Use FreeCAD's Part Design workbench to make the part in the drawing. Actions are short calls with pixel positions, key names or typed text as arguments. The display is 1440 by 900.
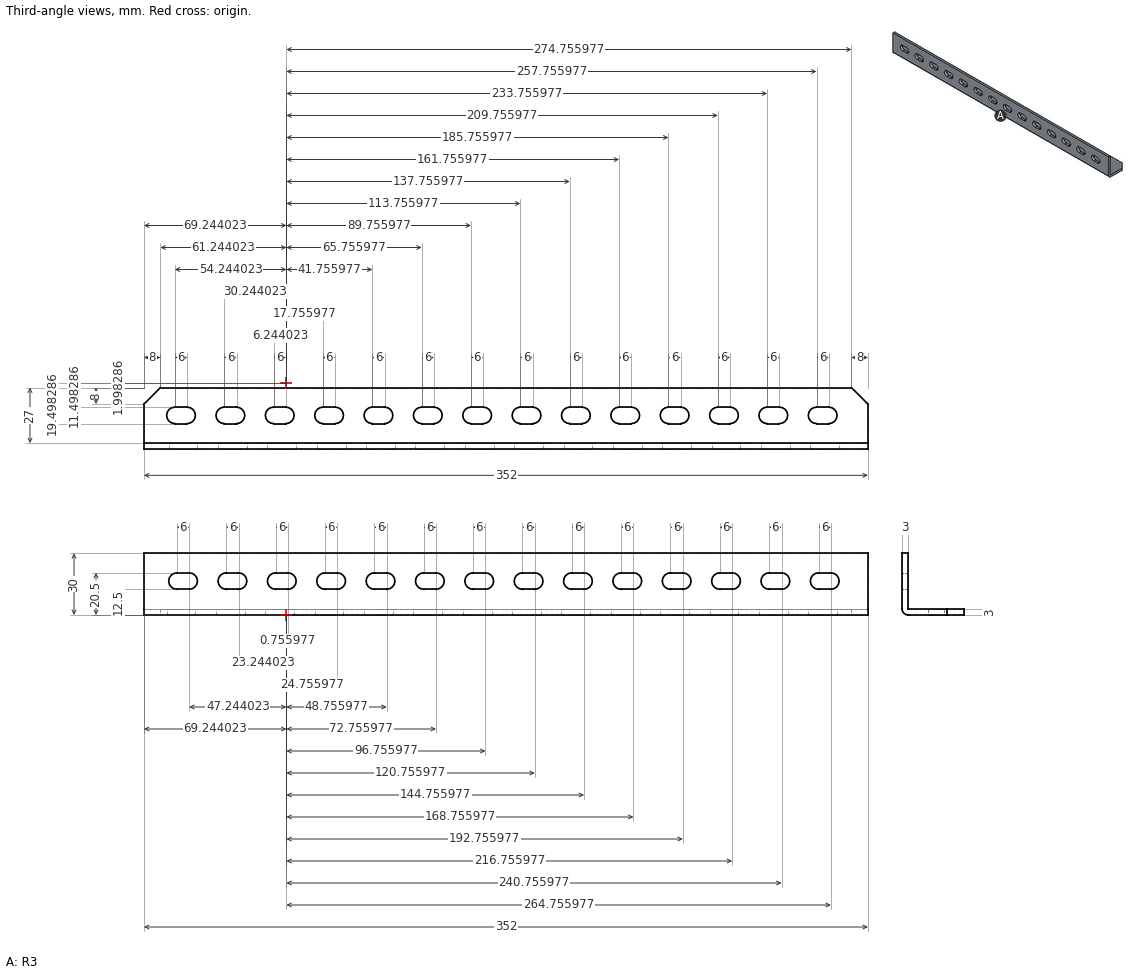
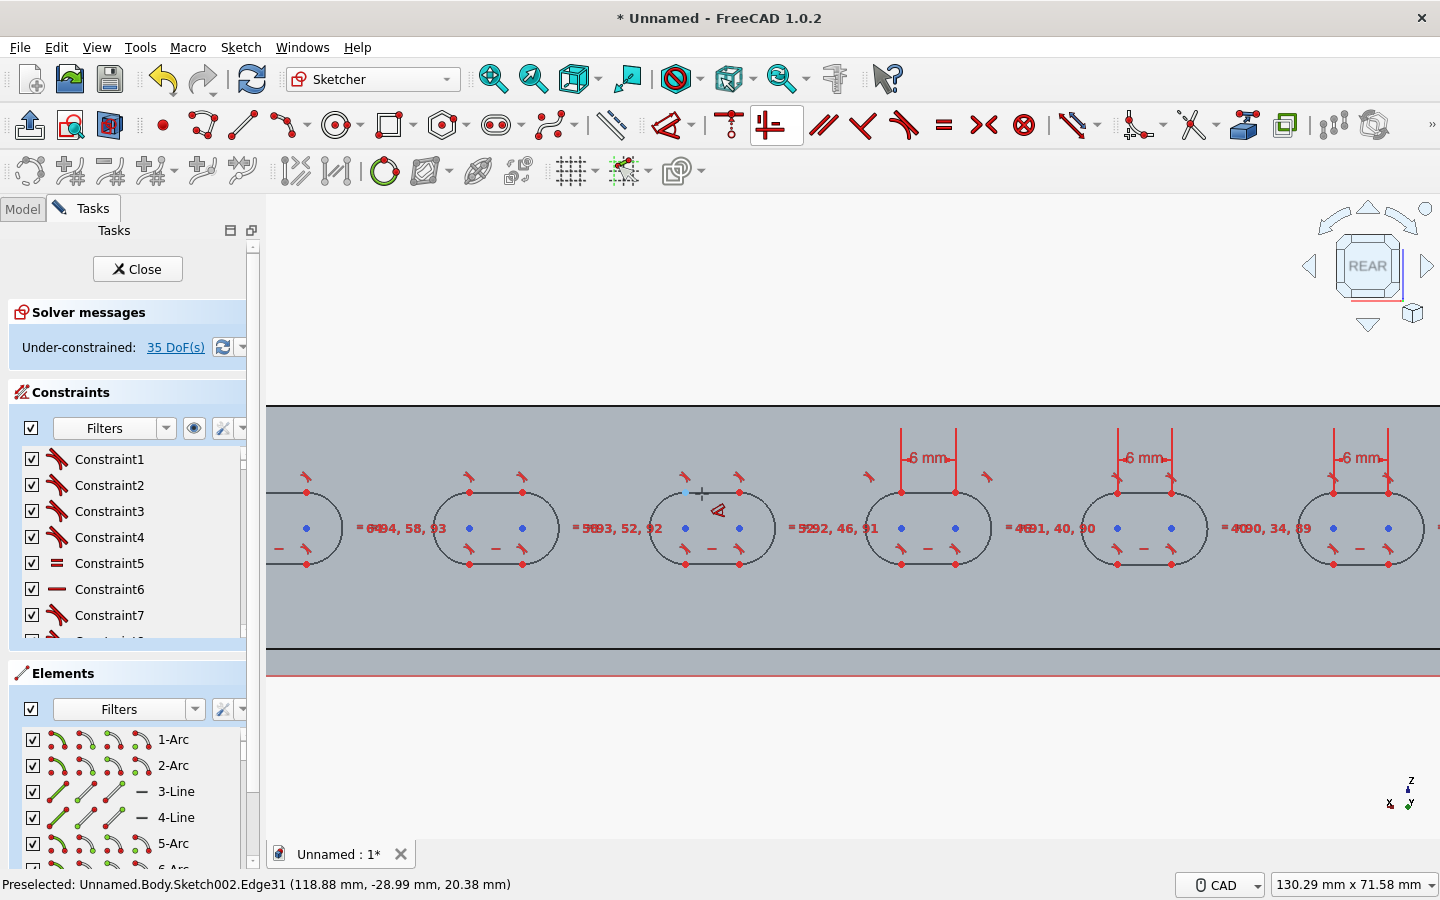
click(702, 493)
click(712, 459)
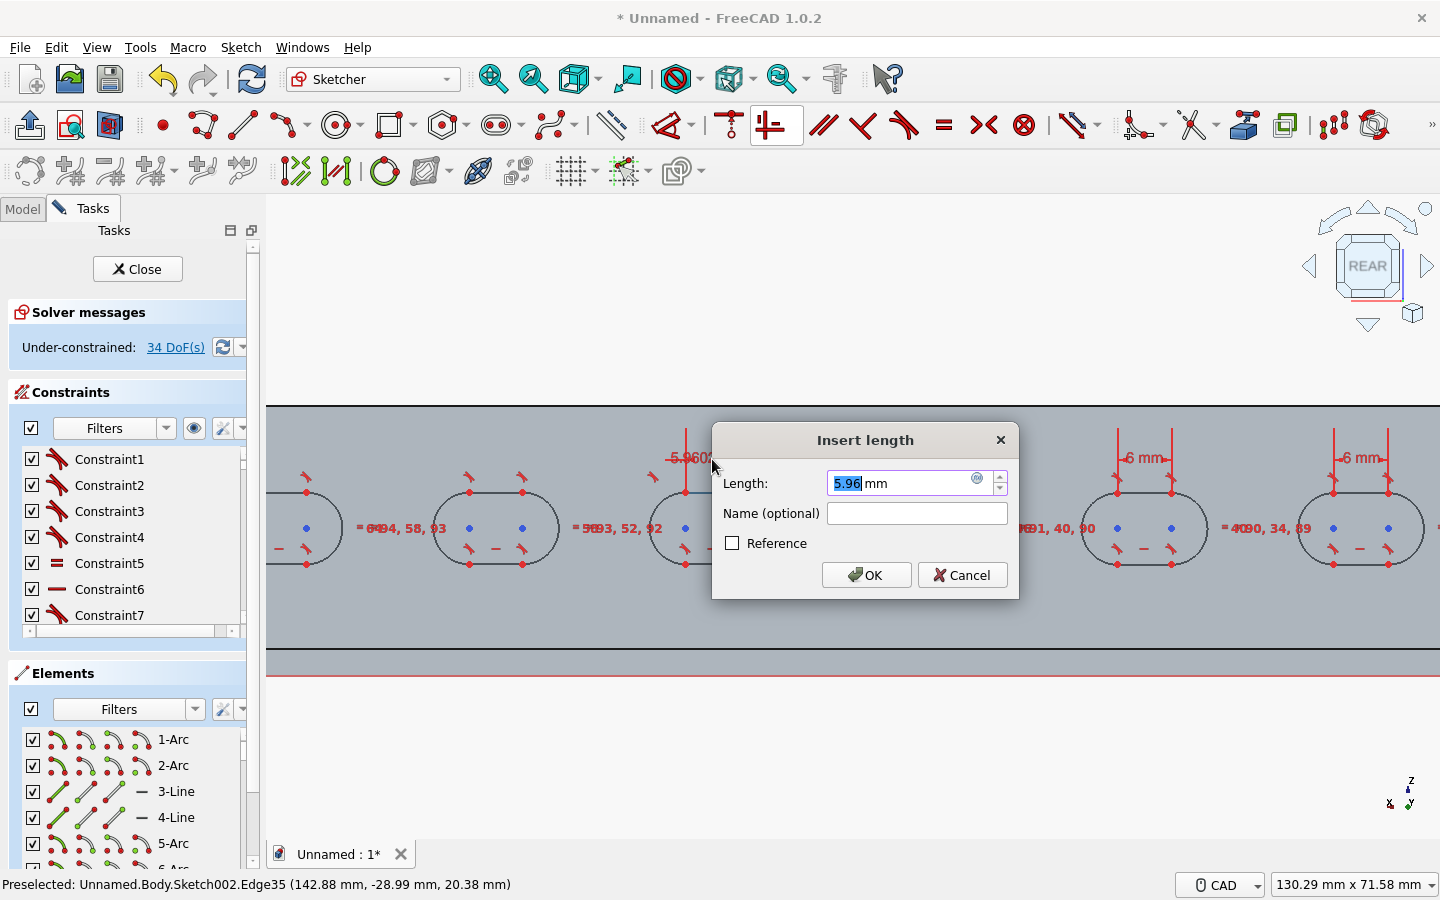
text(6)
key(Return)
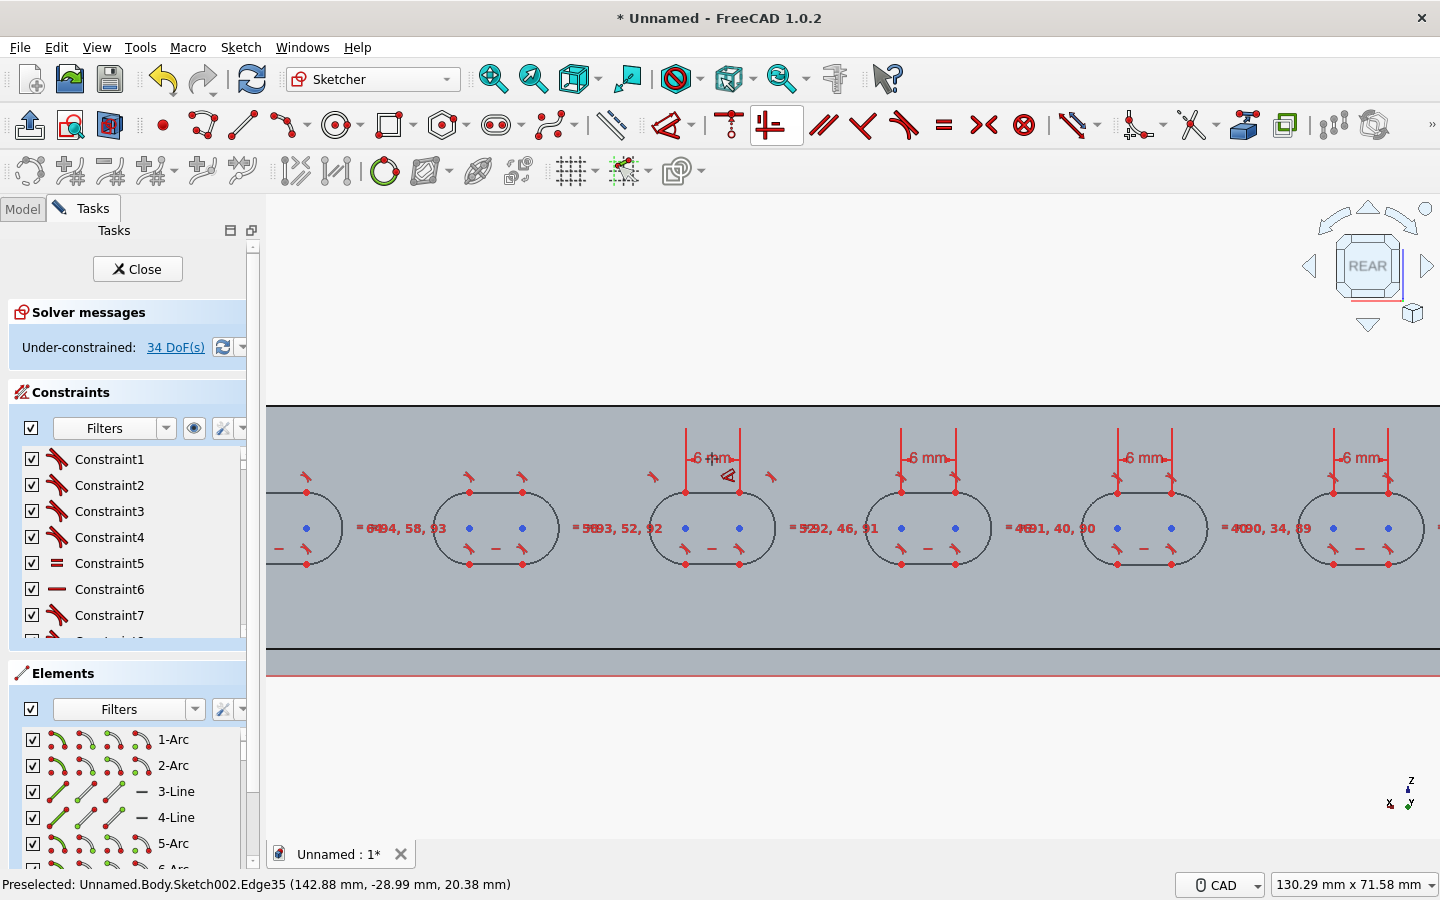
click(485, 493)
click(496, 459)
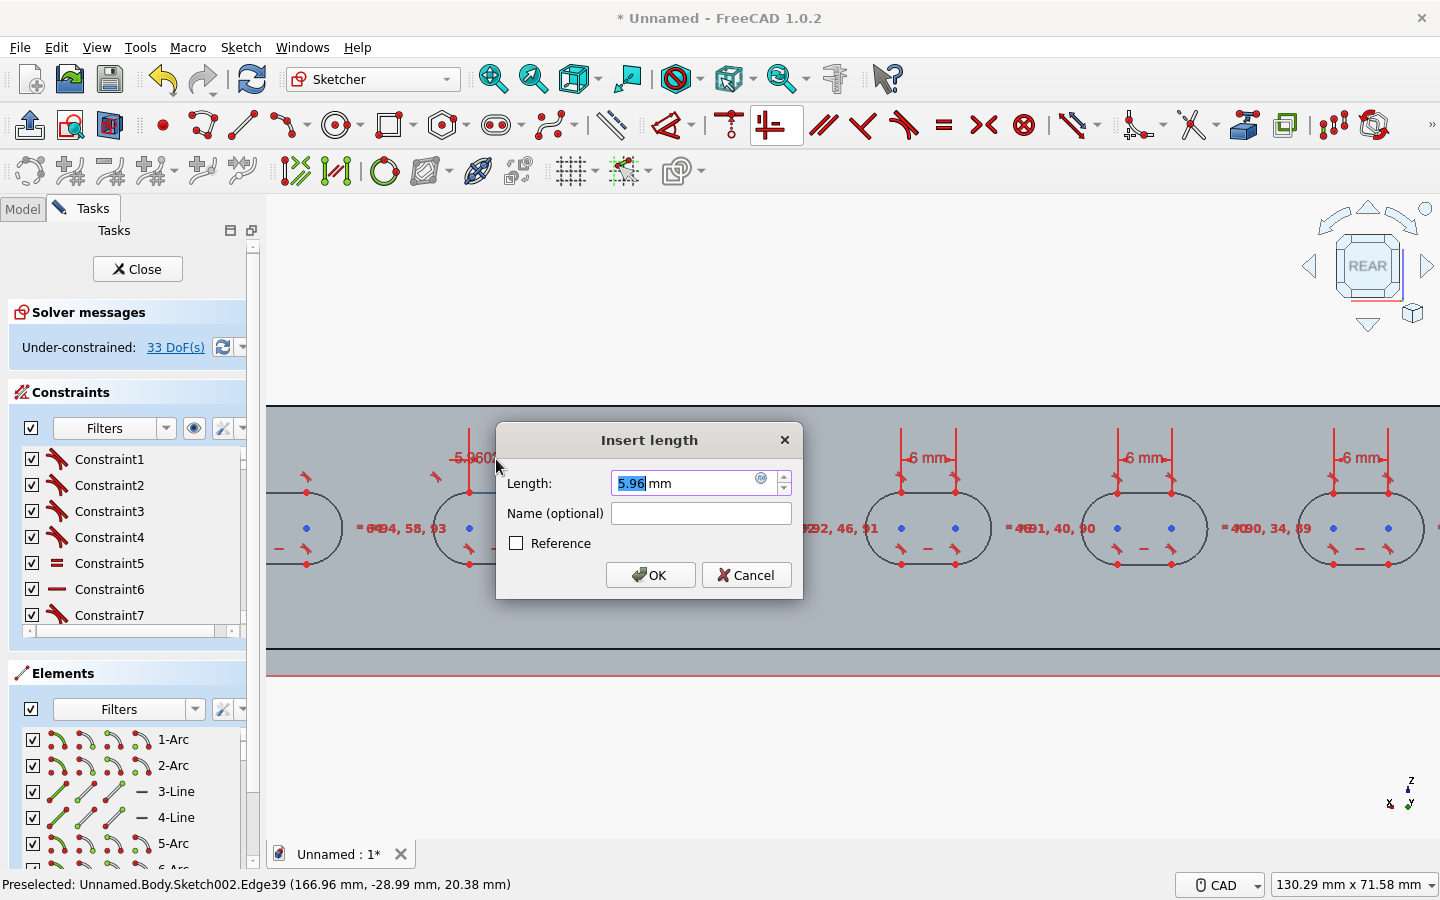
text(6)
key(Return)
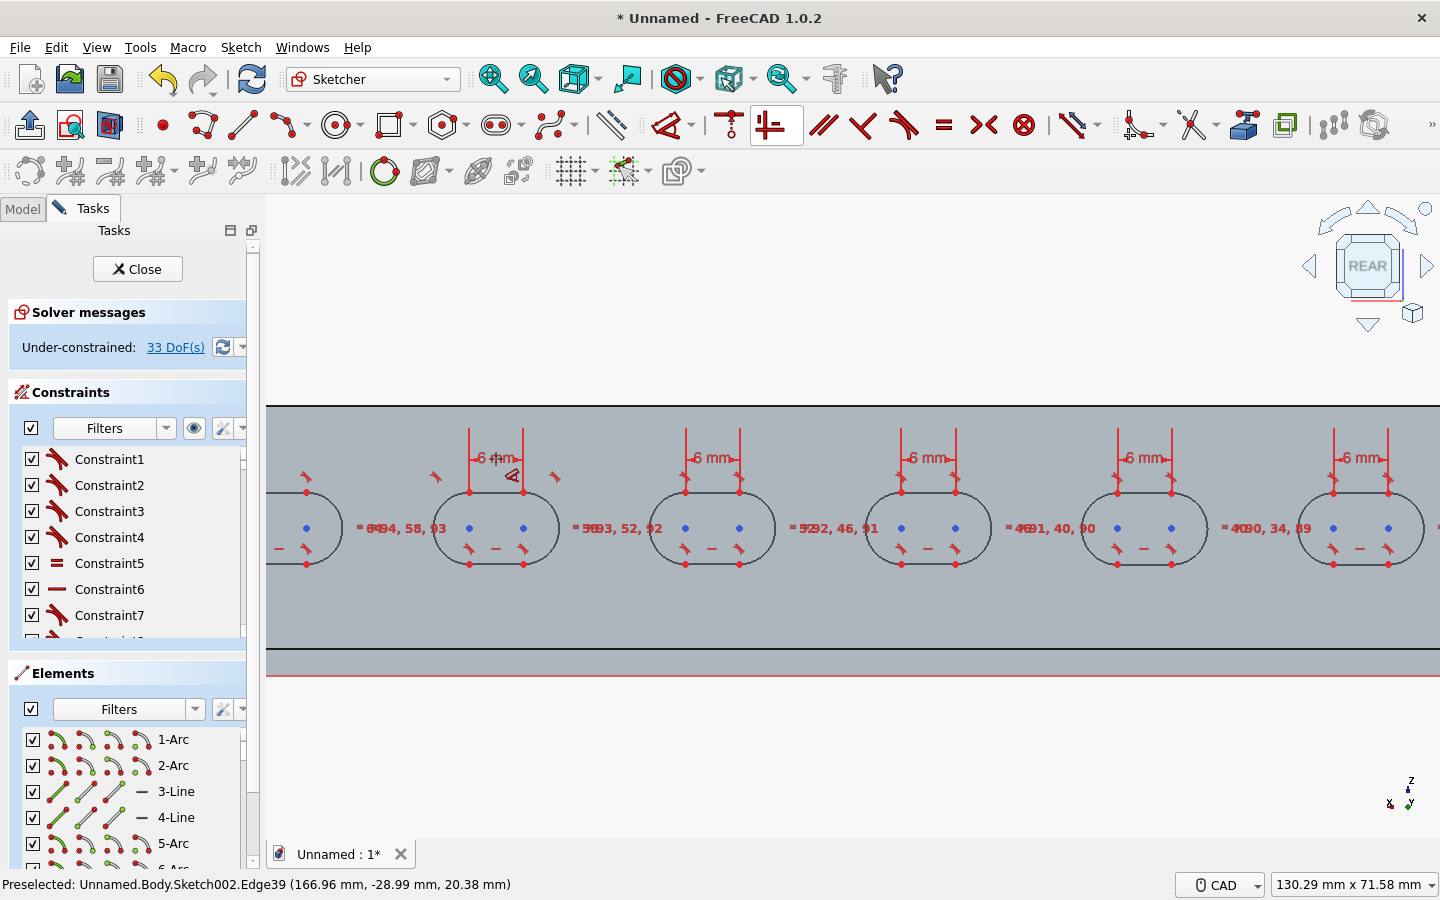
scroll(296, 493, up, 2)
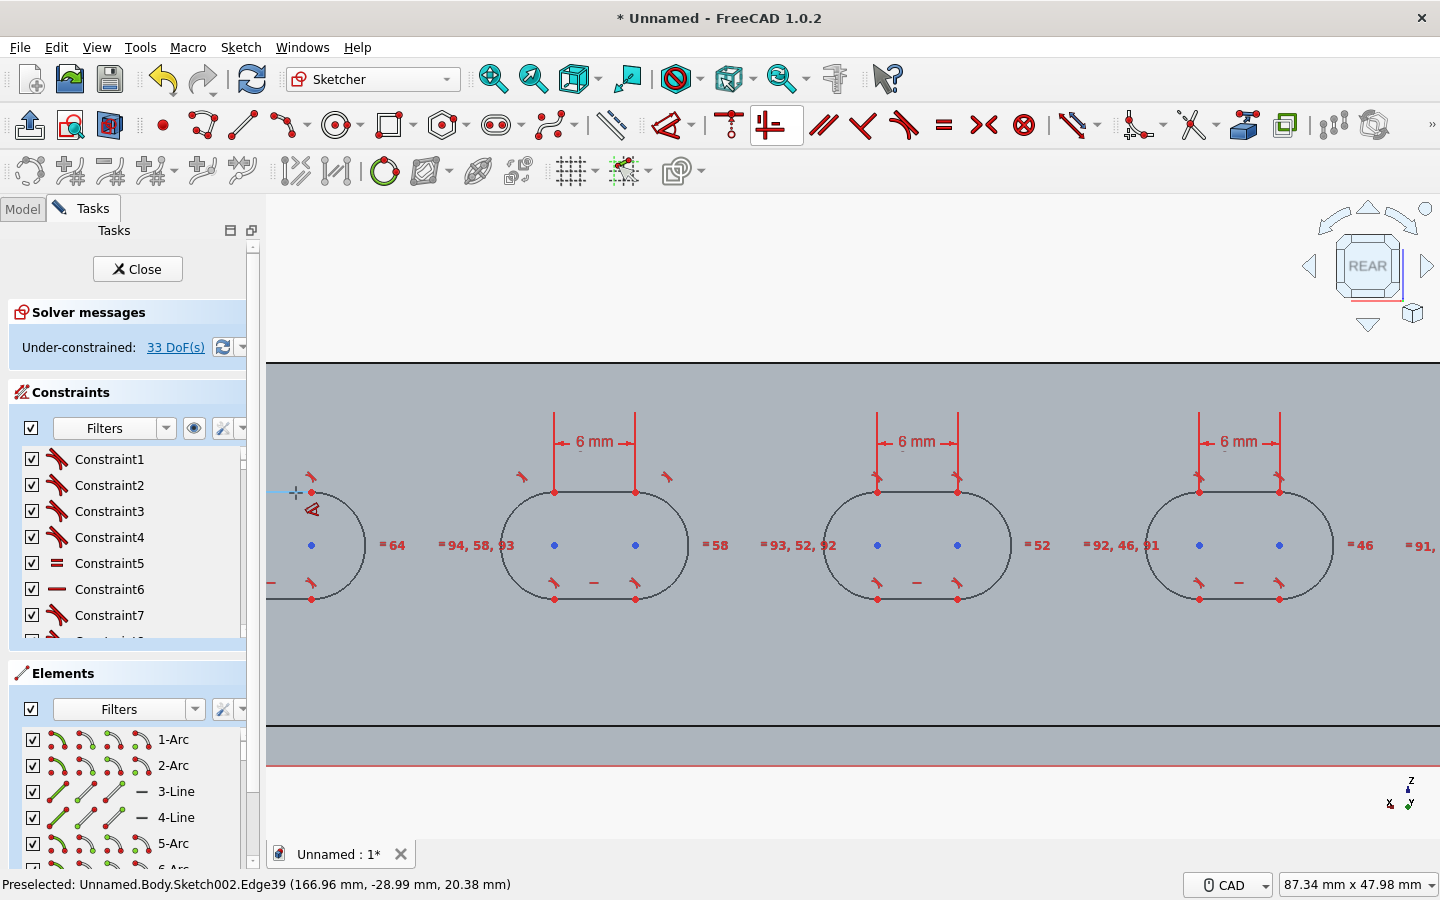
click(296, 492)
click(303, 458)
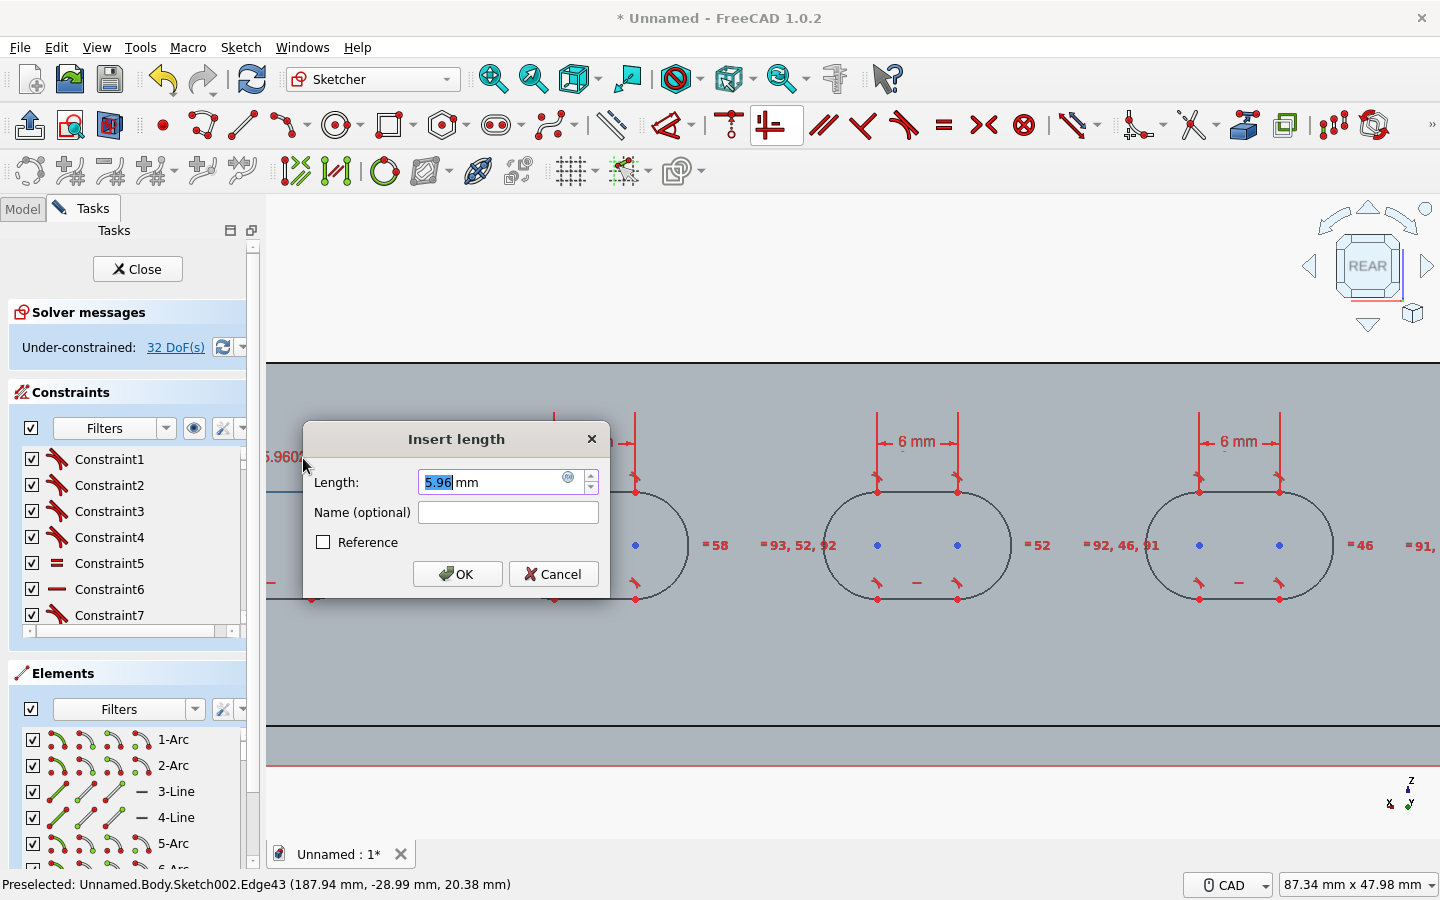
text(6)
key(Return)